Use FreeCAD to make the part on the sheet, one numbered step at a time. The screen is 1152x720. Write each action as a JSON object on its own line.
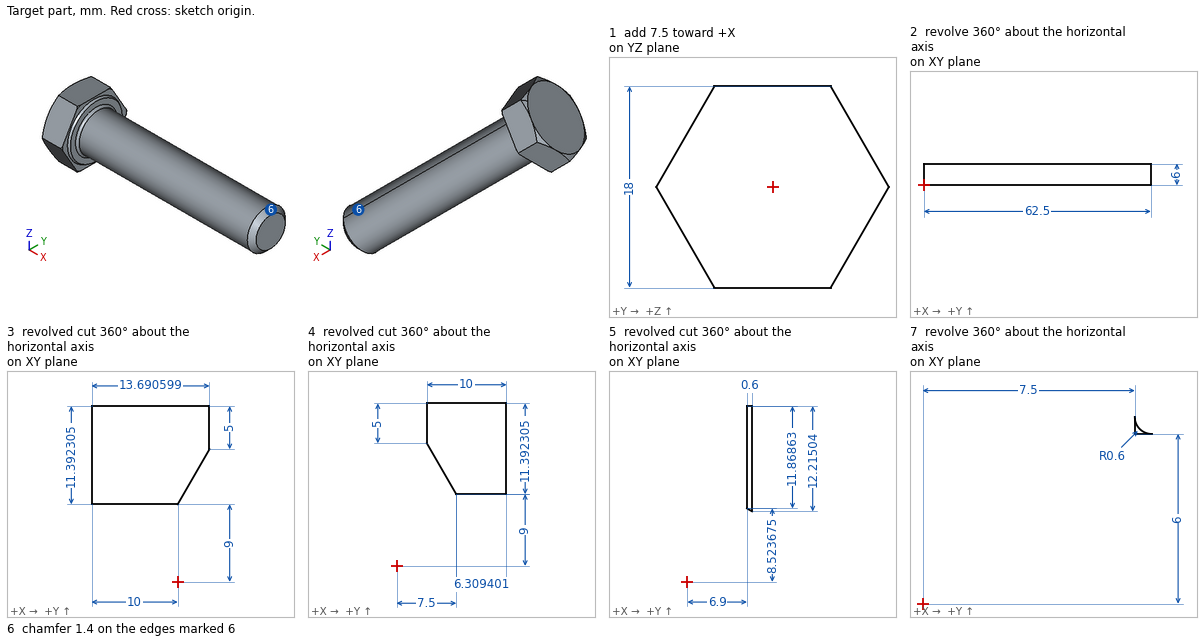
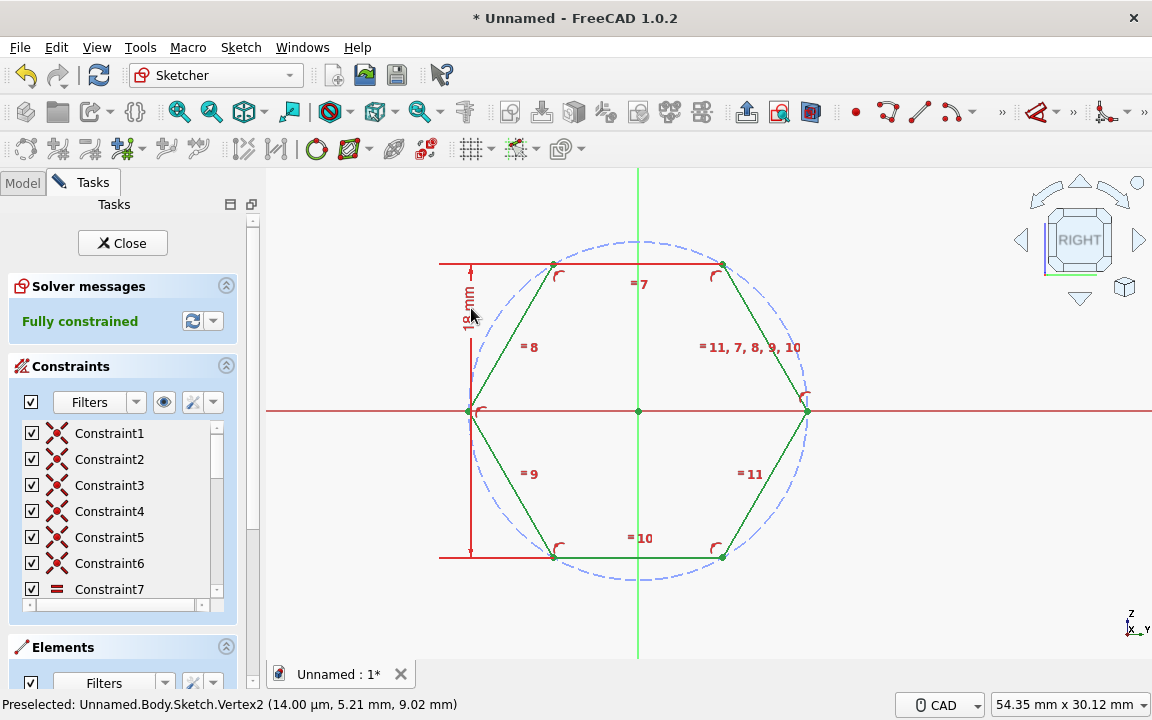
{"action": "left_click", "coordinate": [123, 243]}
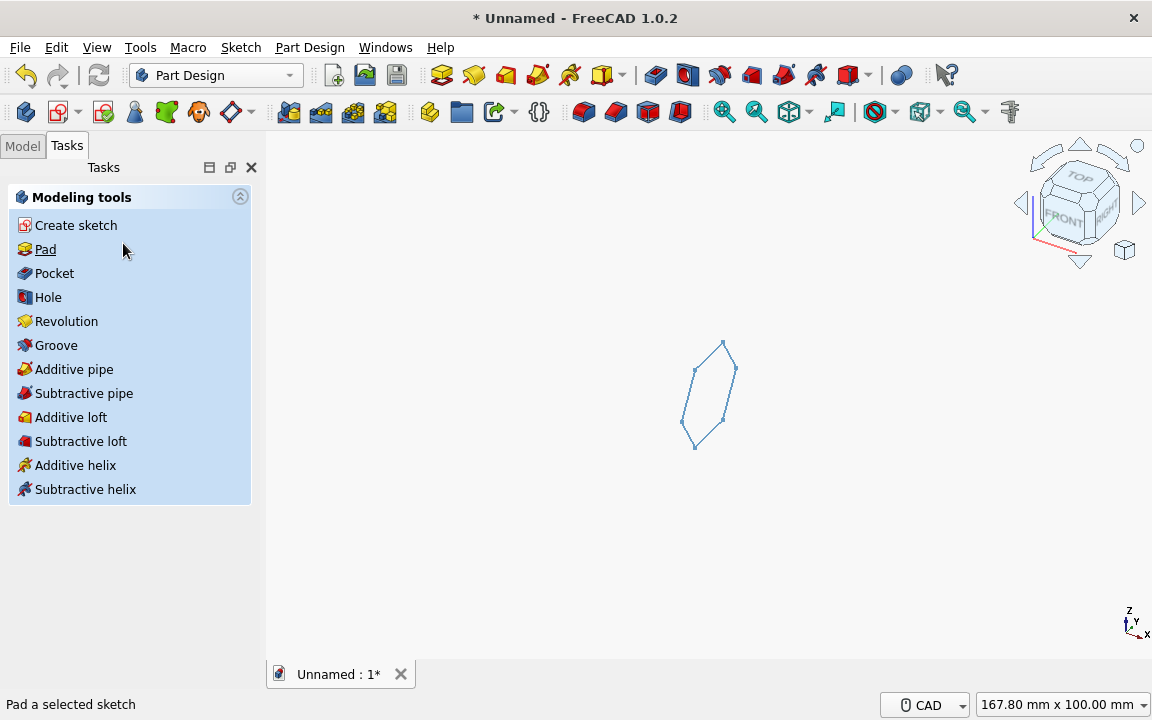
{"action": "left_click", "coordinate": [442, 76]}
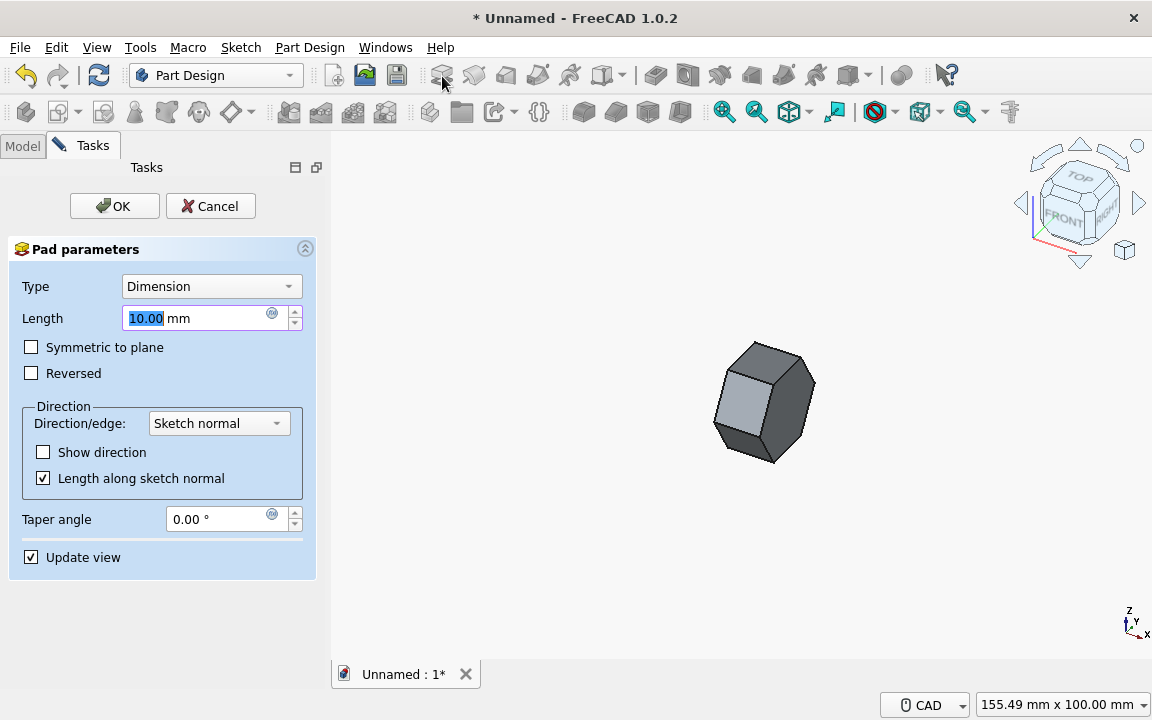
{"action": "type", "text": "7.5"}
{"action": "key", "text": "Tab"}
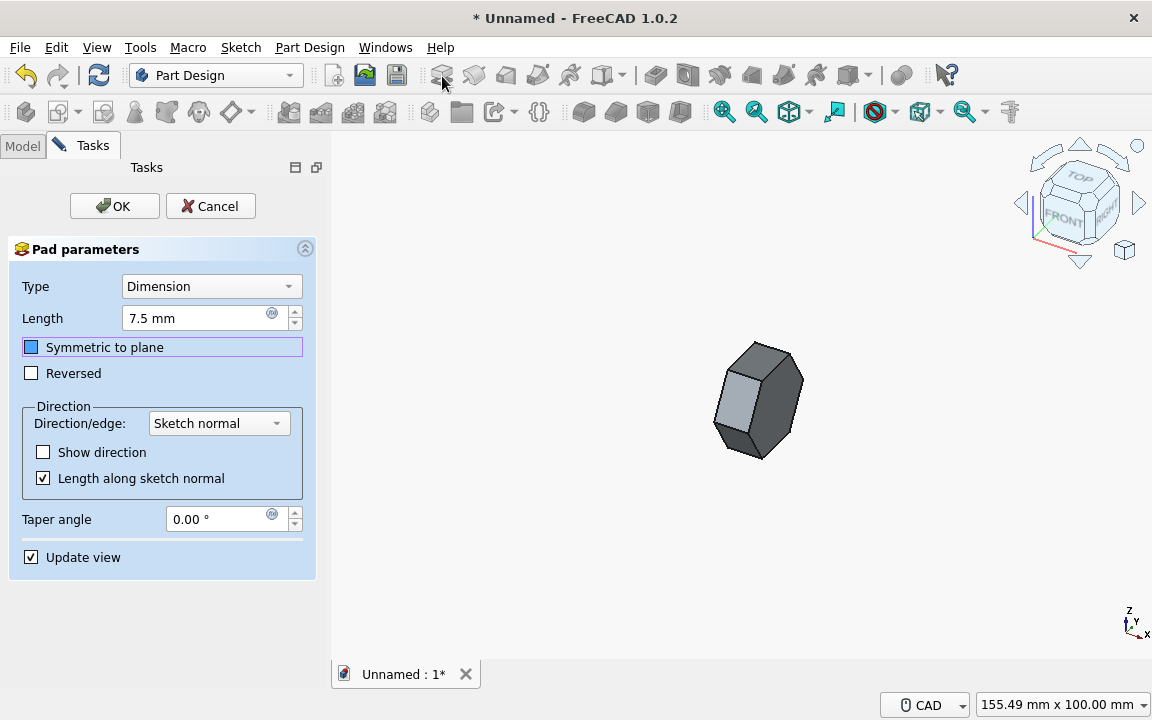
{"action": "left_click", "coordinate": [115, 206]}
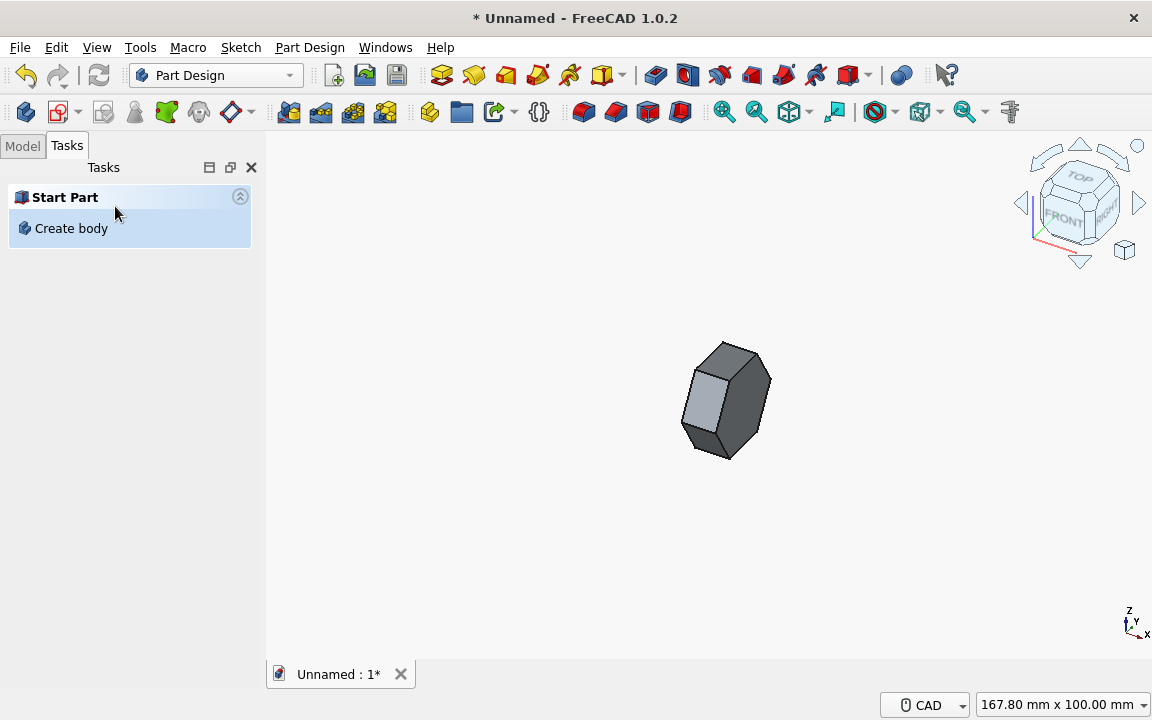
{"action": "key", "text": "v f"}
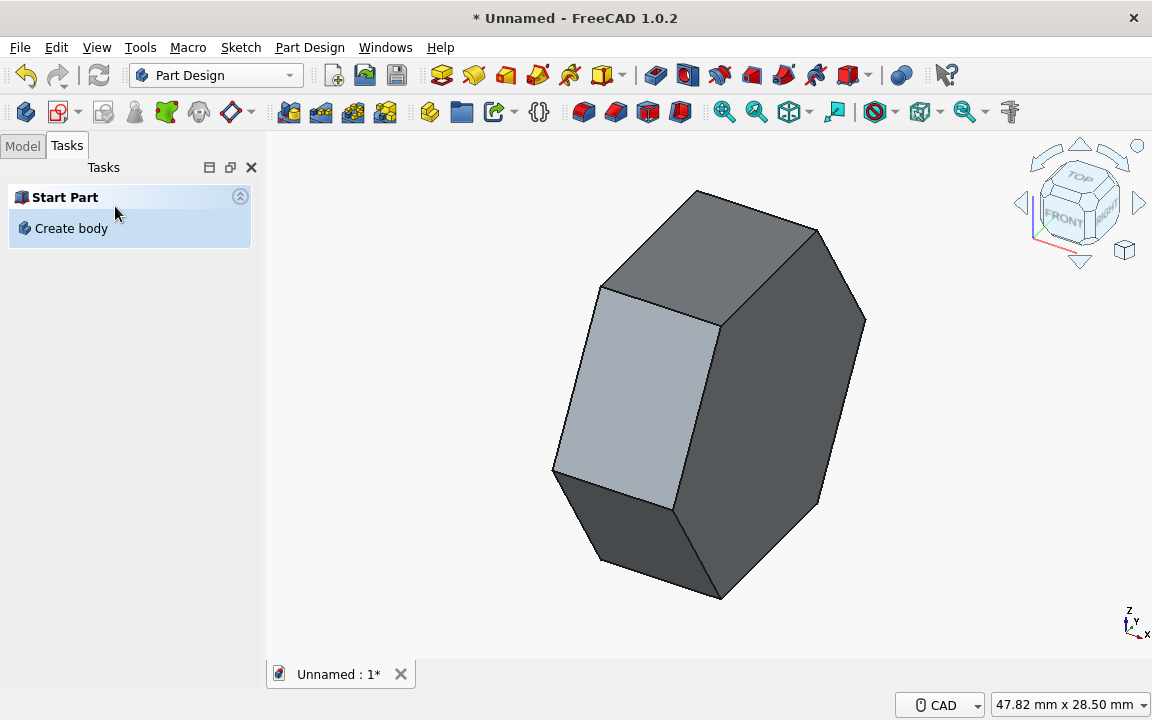
{"action": "left_click", "coordinate": [58, 112]}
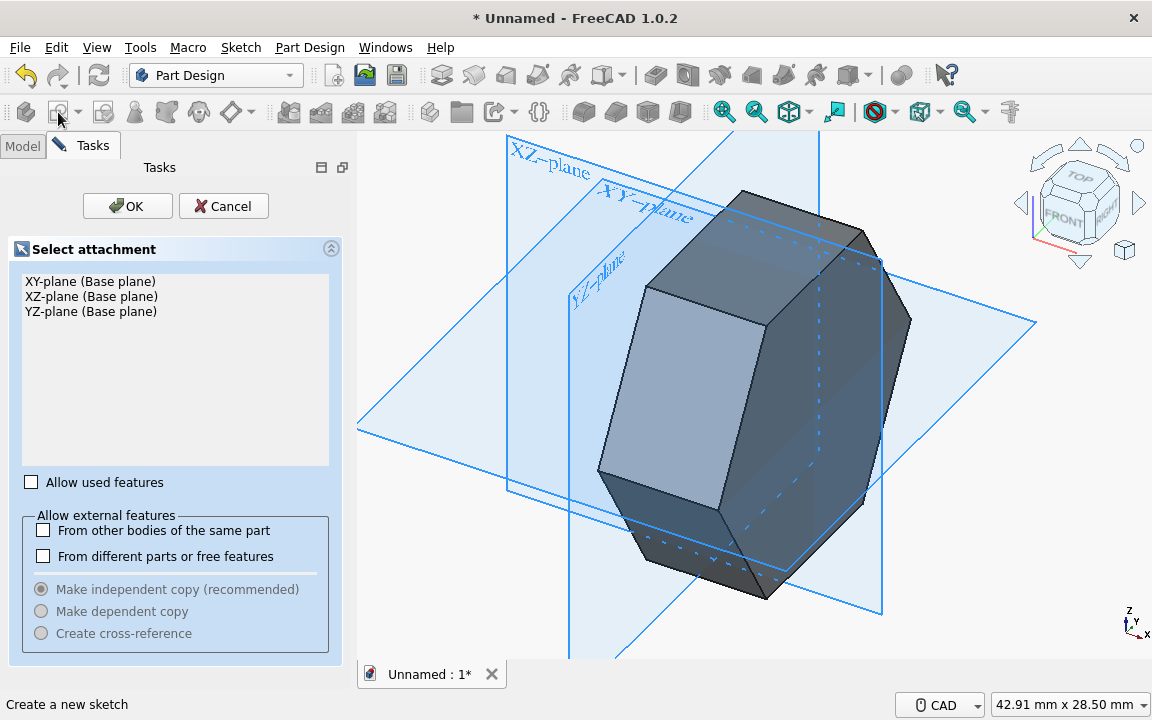
{"action": "left_click", "coordinate": [82, 282]}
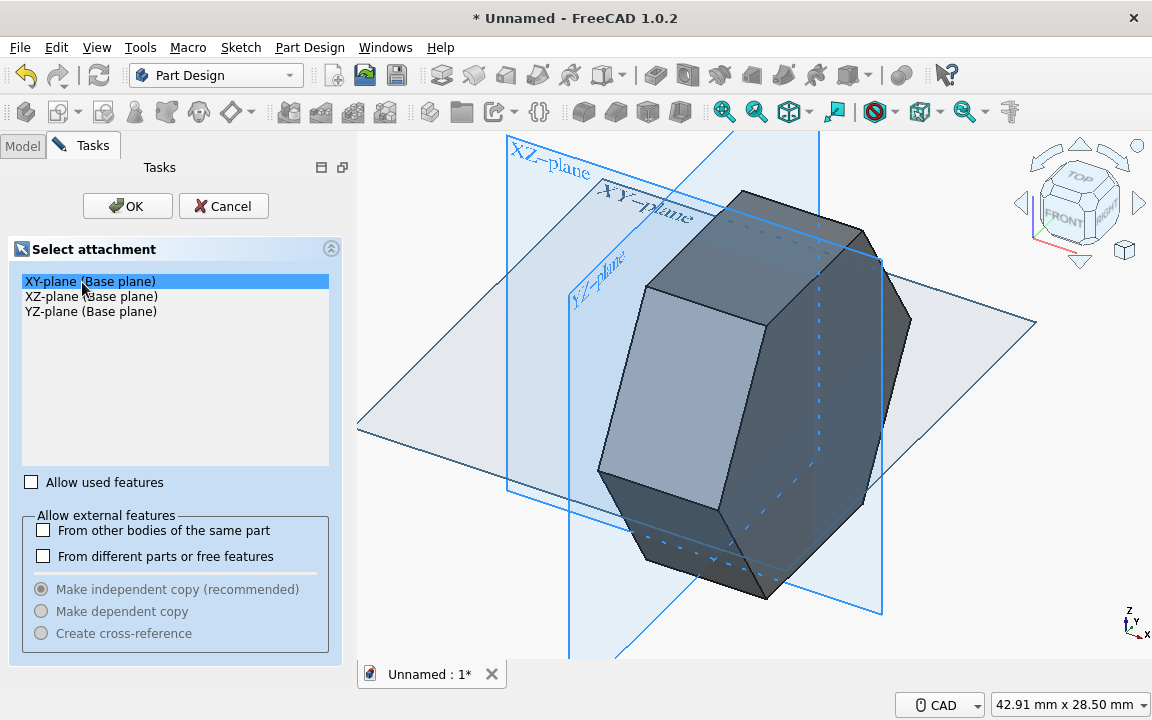
{"action": "left_click", "coordinate": [128, 206]}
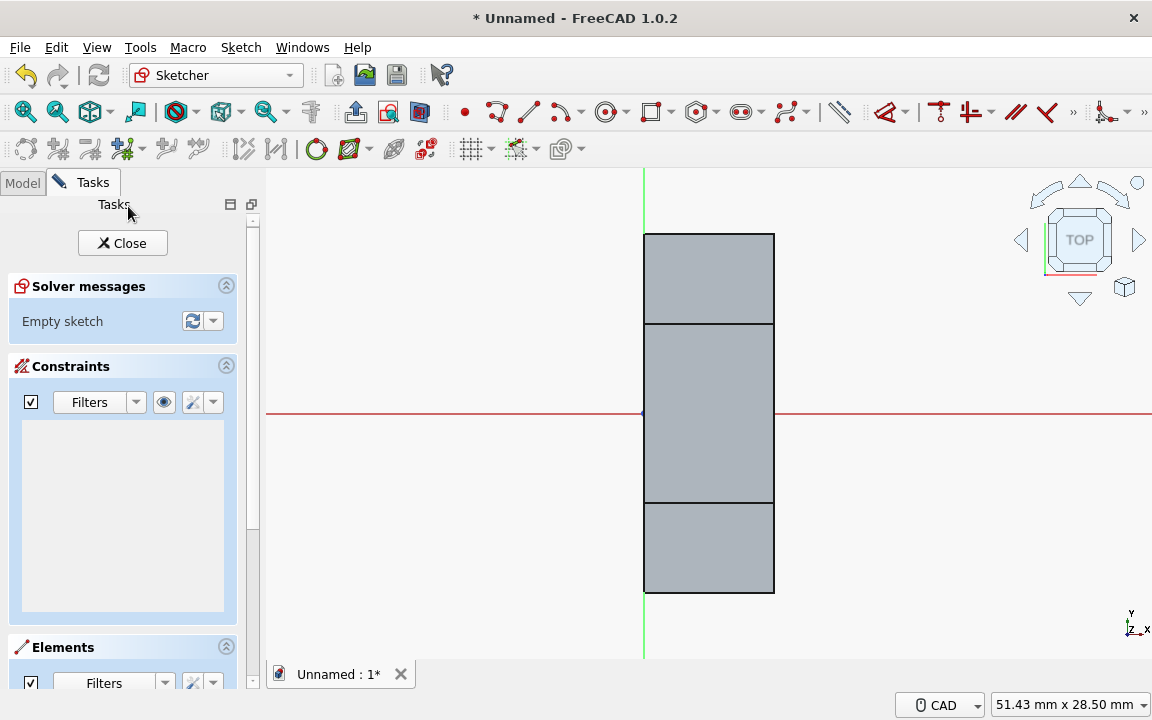
{"action": "key", "text": "q s"}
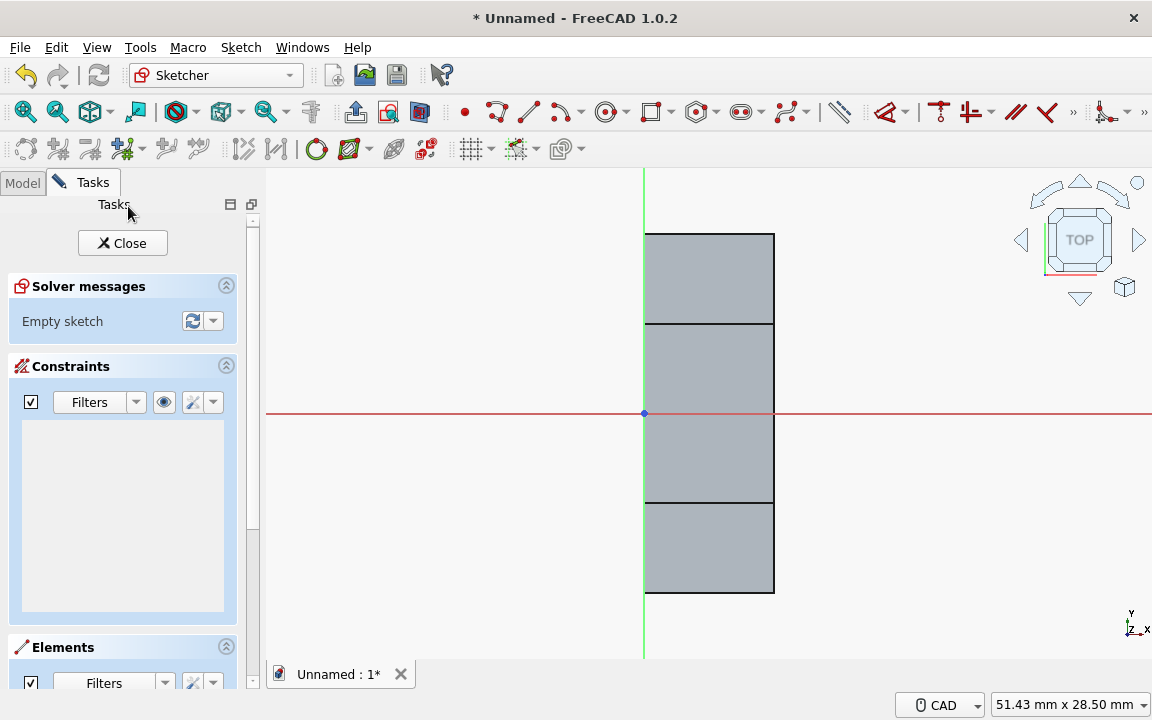
{"action": "scroll", "coordinate": [294, 456], "scroll_direction": "down", "scroll_amount": 4}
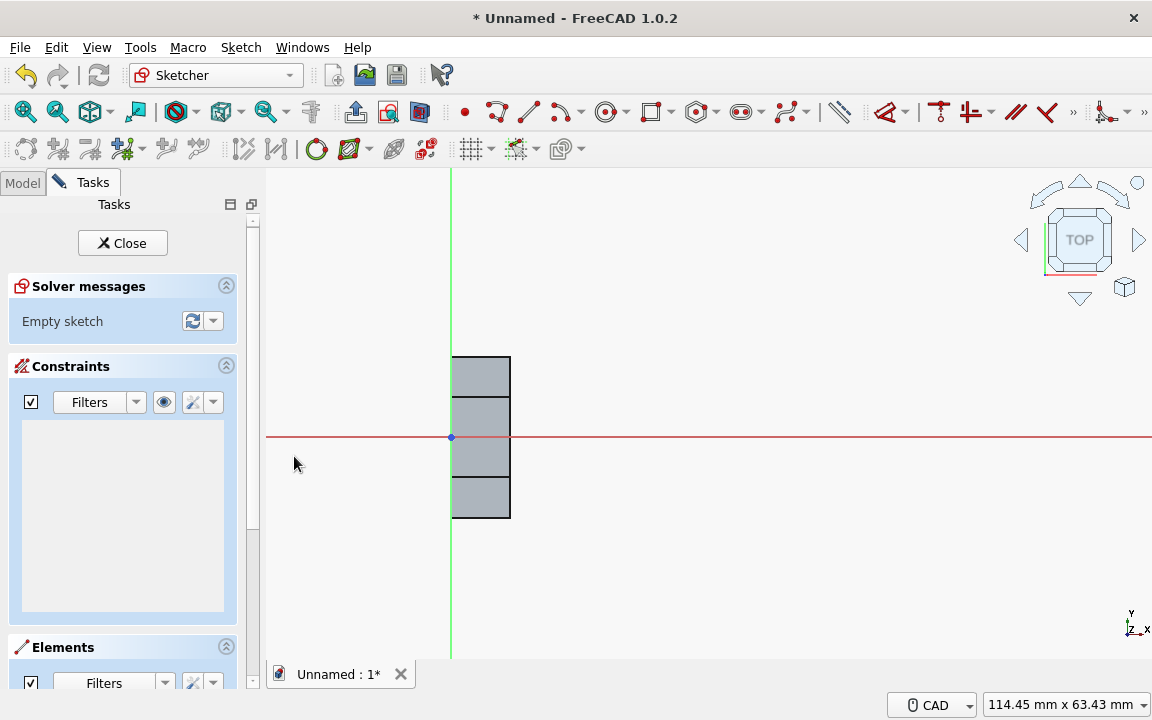
{"action": "left_click", "coordinate": [652, 112]}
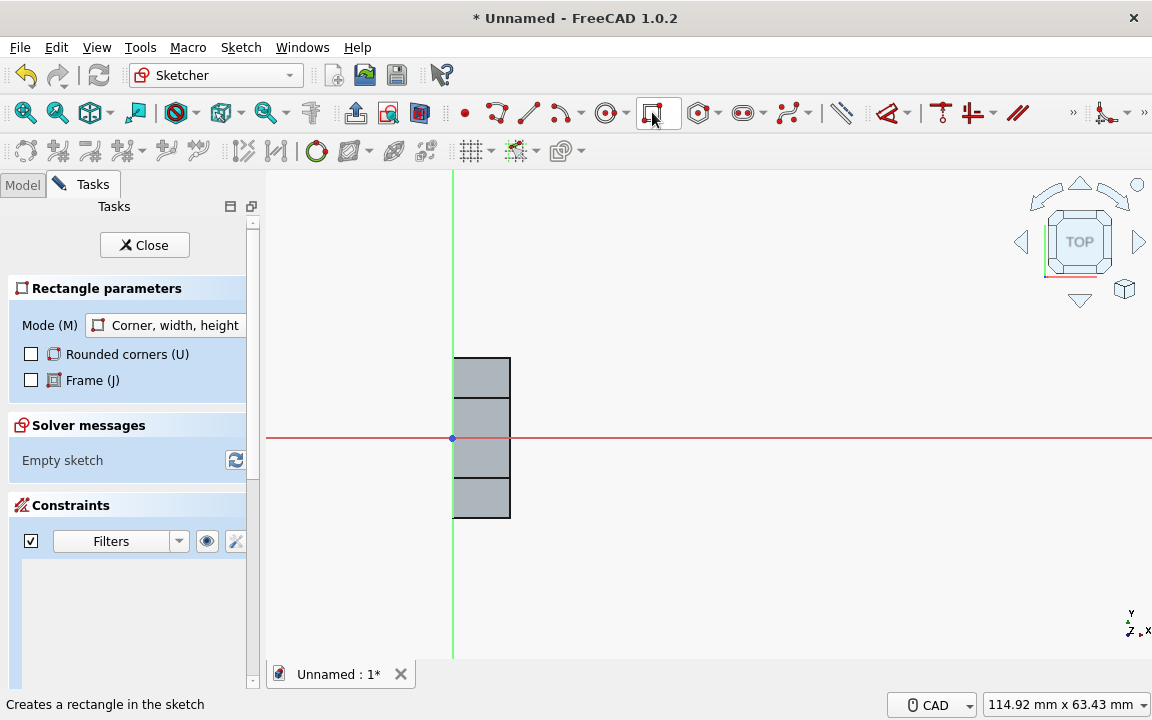
{"action": "left_click", "coordinate": [453, 438]}
{"action": "left_click", "coordinate": [934, 392]}
{"action": "key", "text": "Escape"}